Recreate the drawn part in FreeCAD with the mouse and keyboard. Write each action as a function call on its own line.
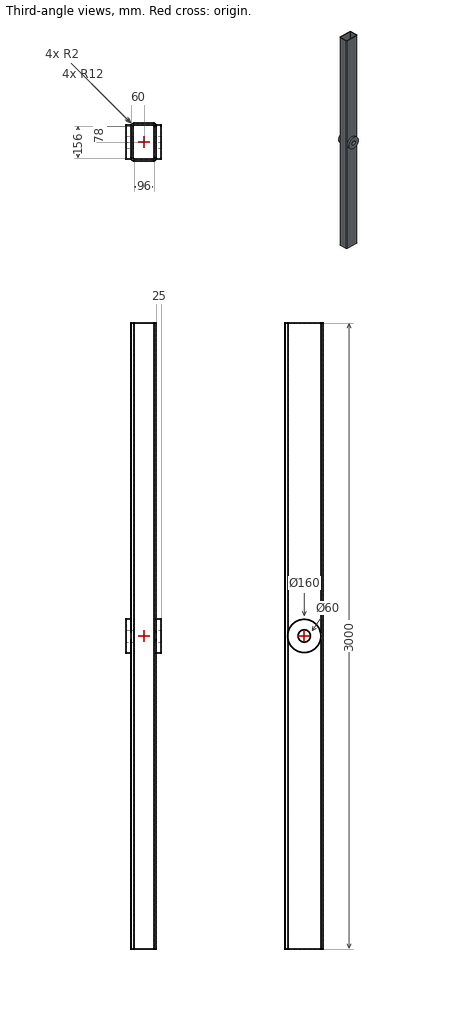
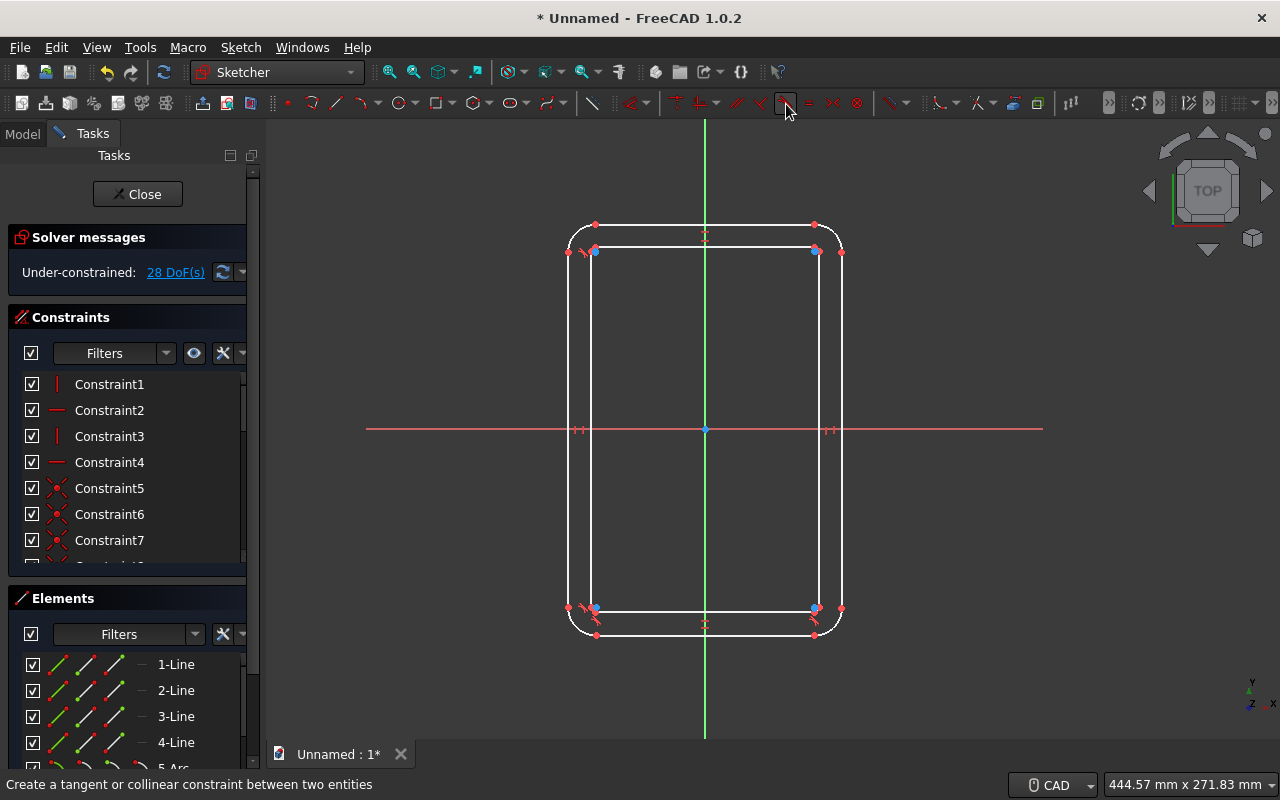
click(842, 502)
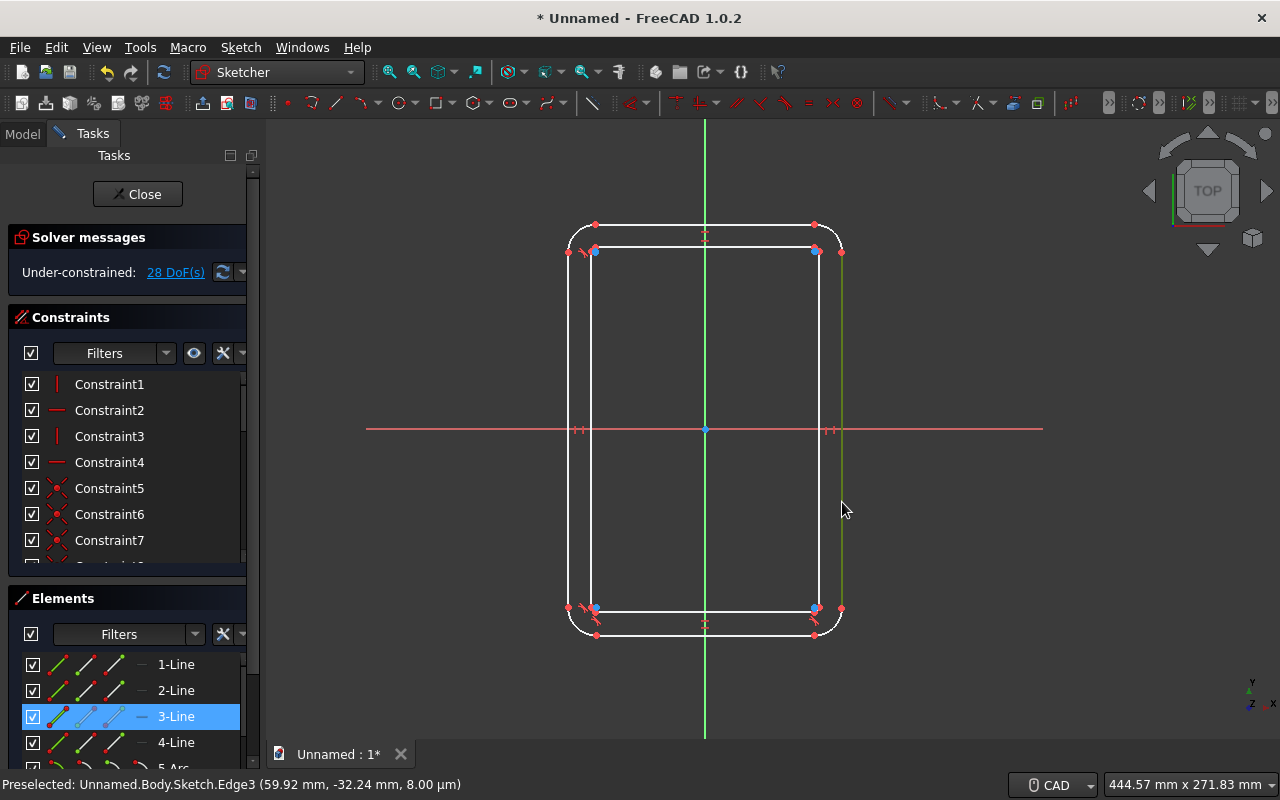
click(827, 633)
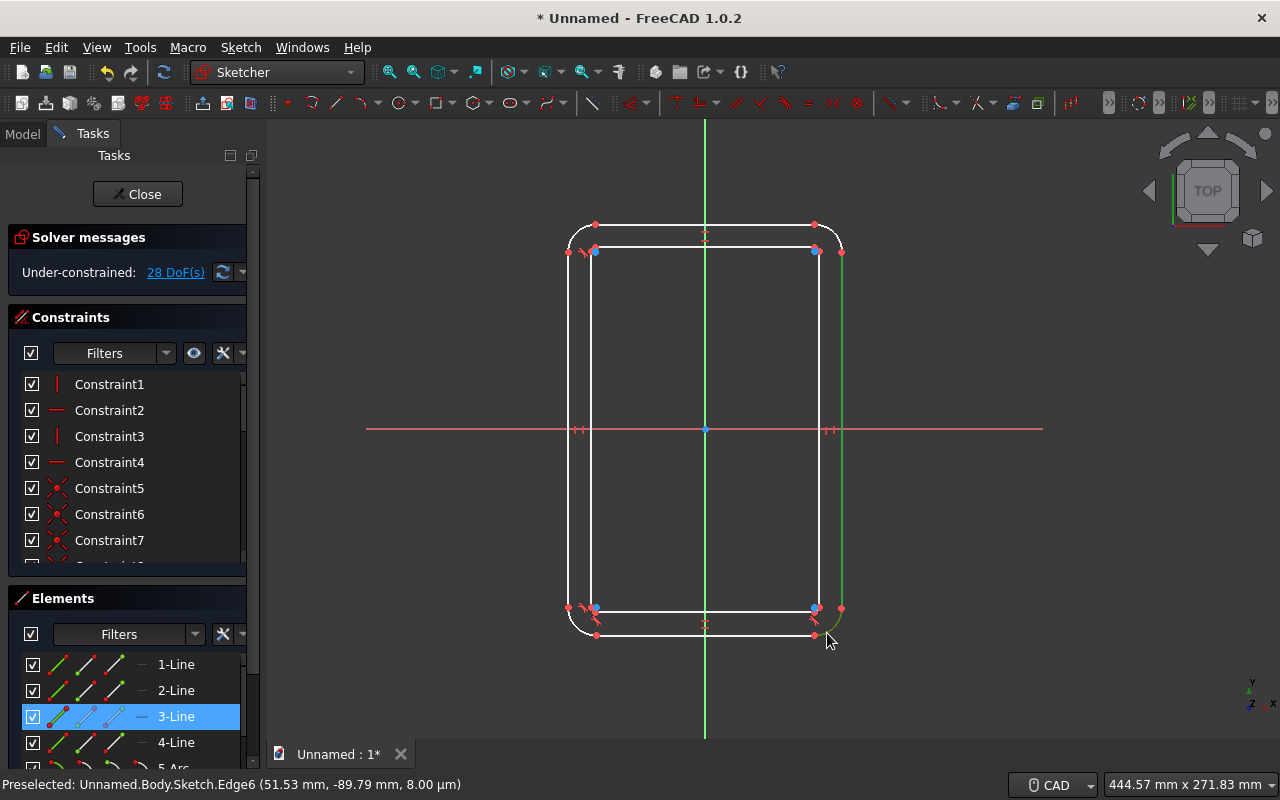
click(786, 104)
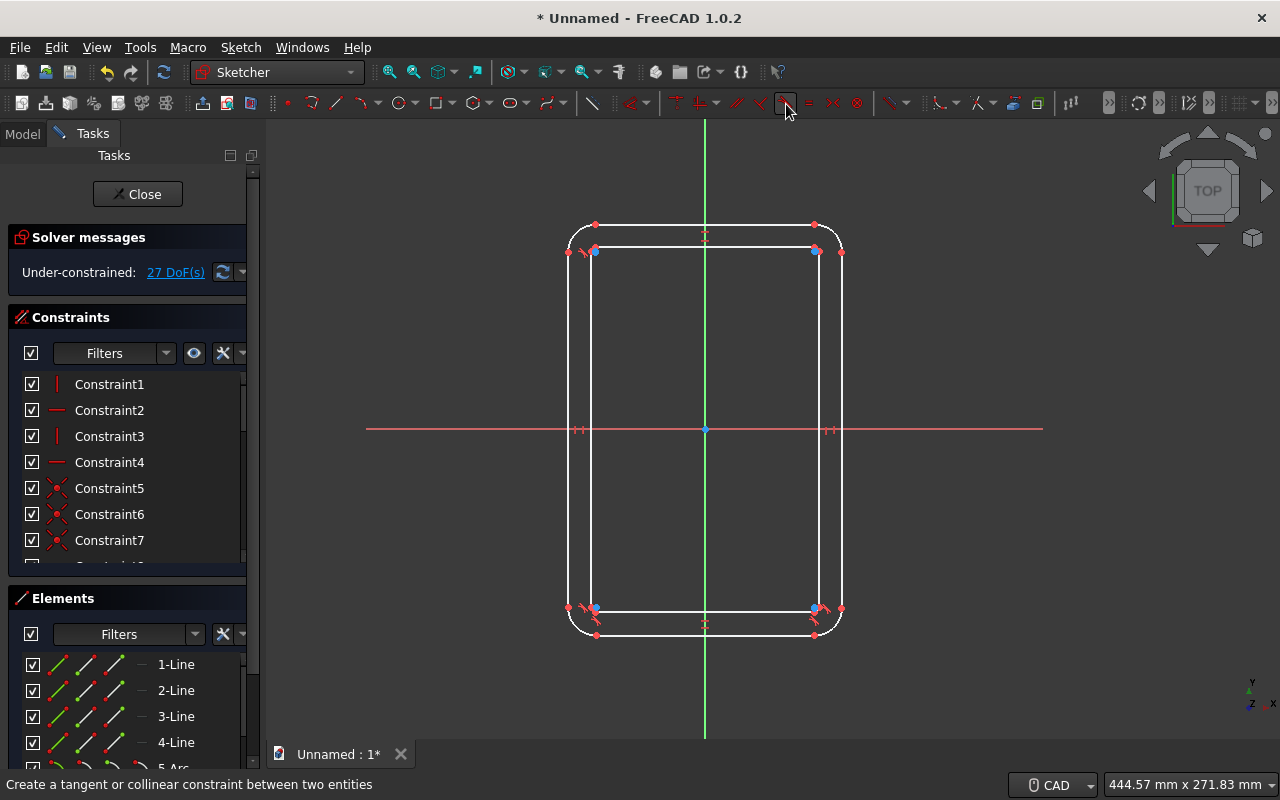
click(842, 501)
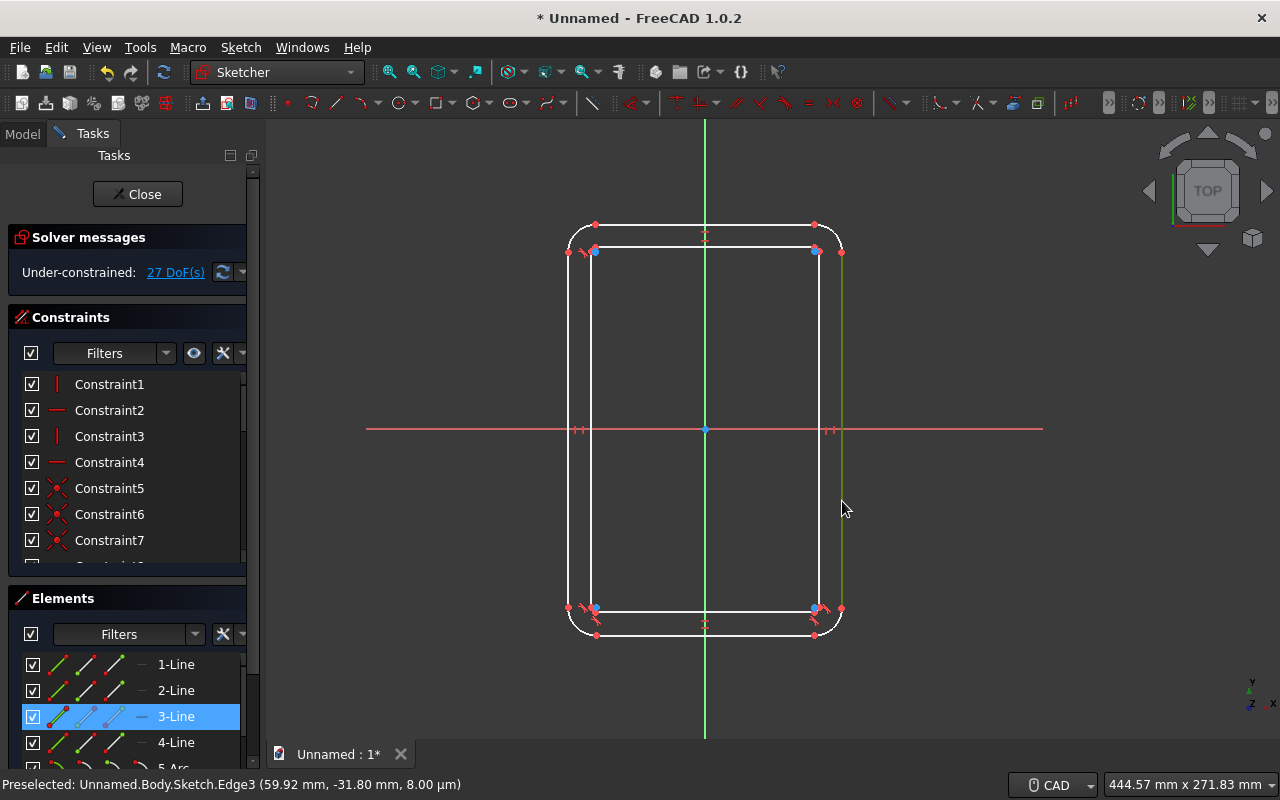
click(839, 240)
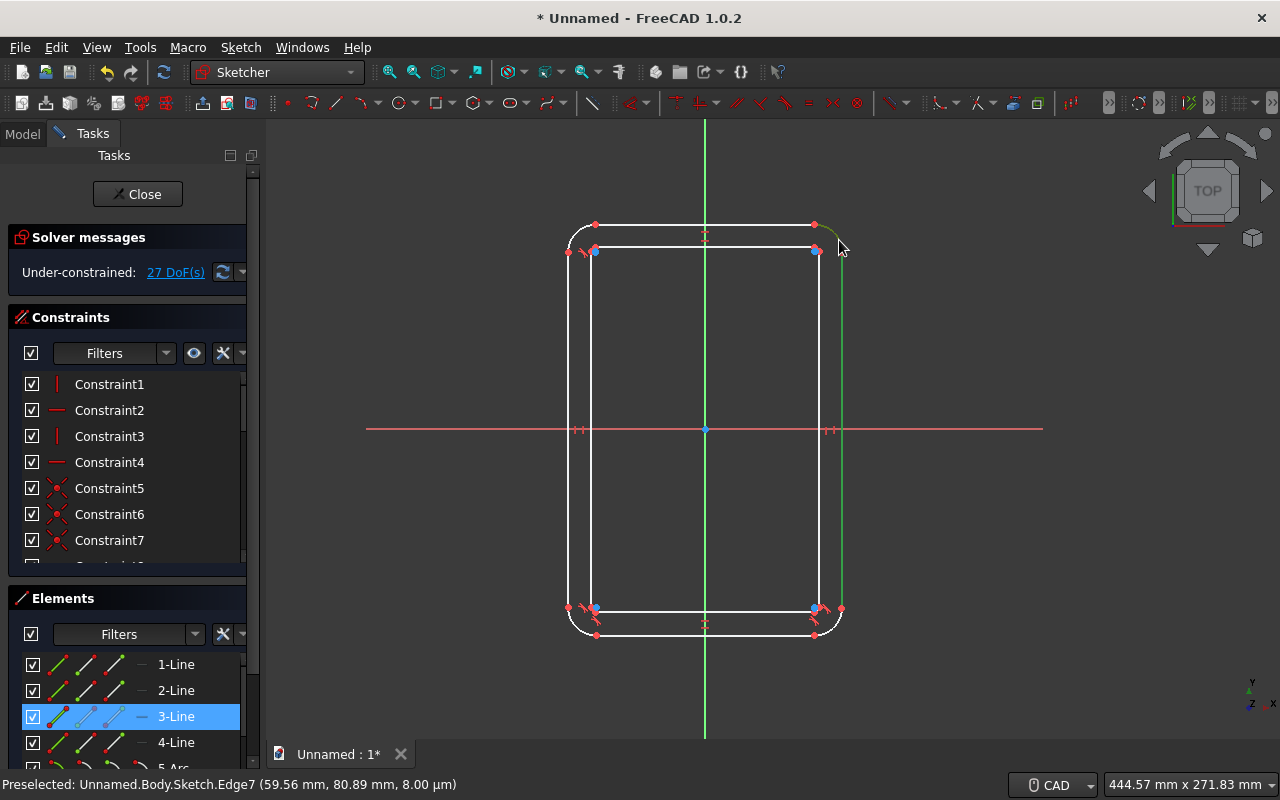
click(786, 104)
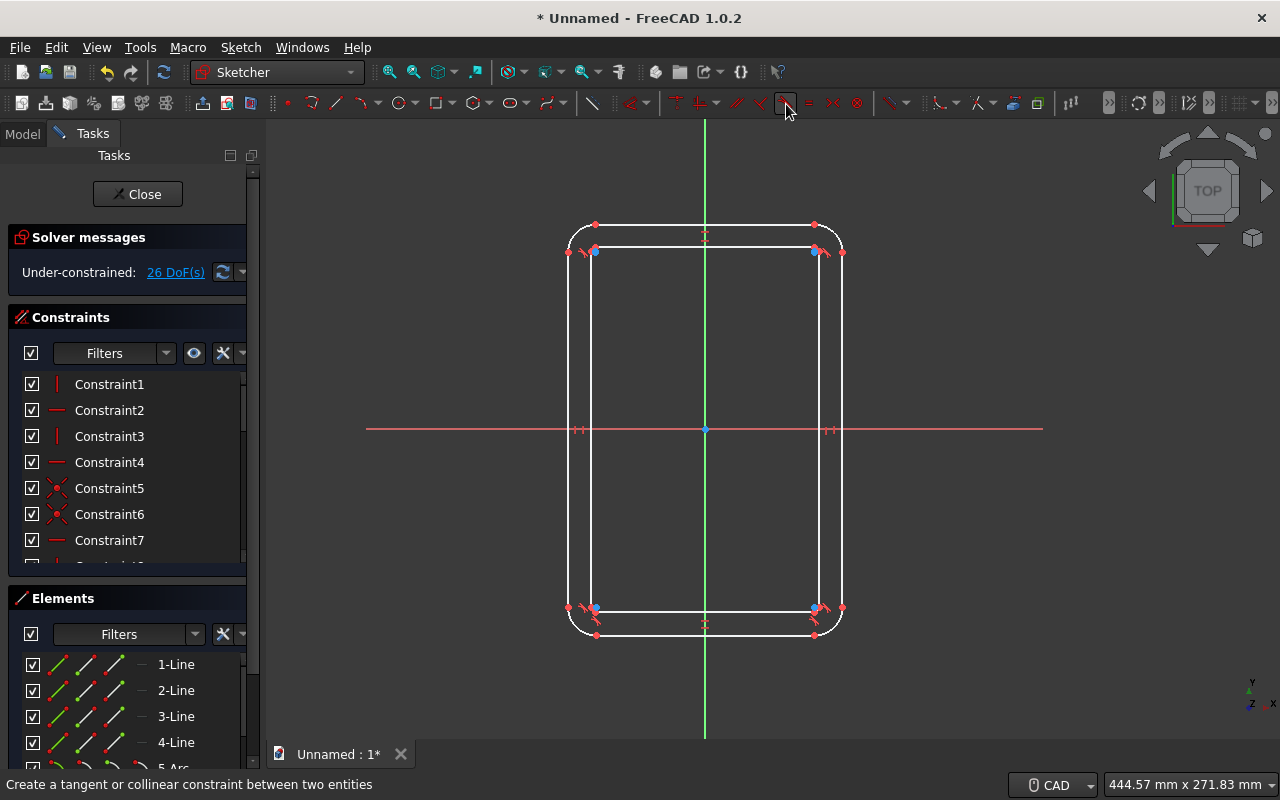
click(749, 225)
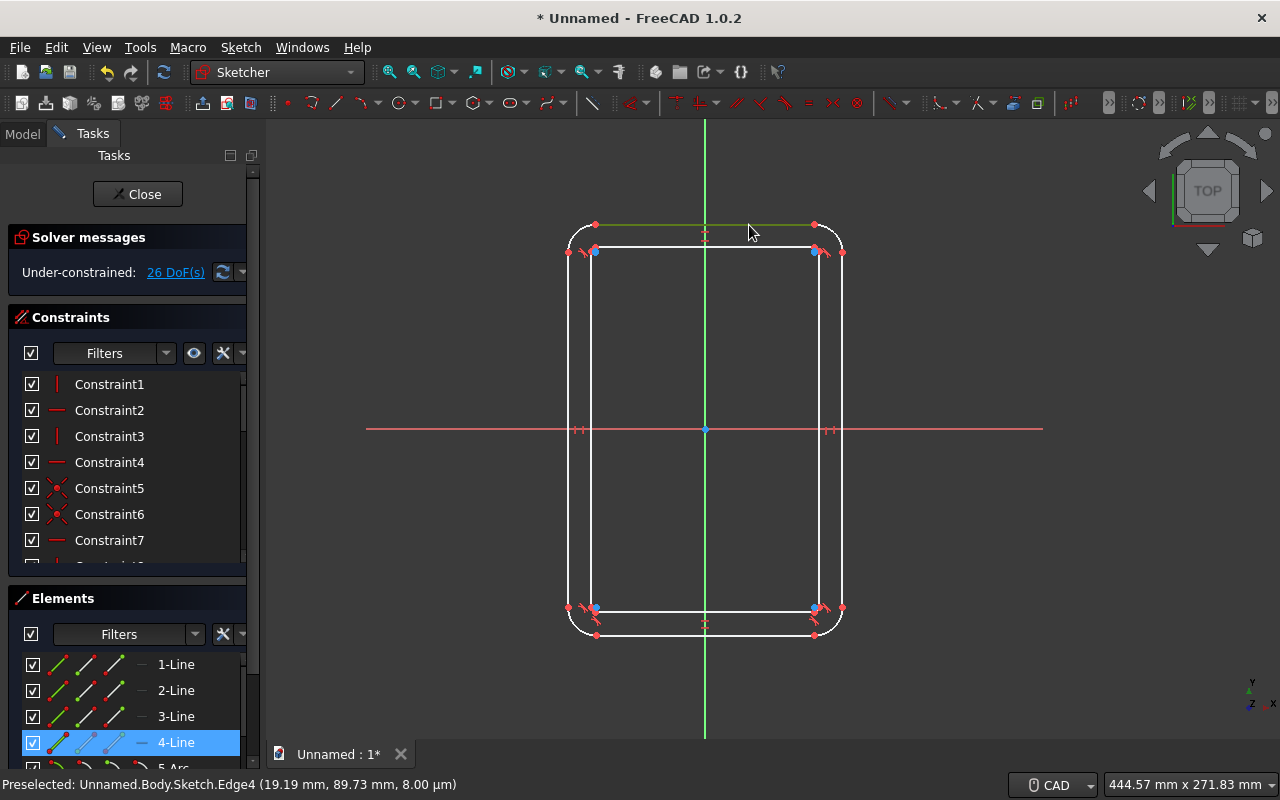
click(839, 240)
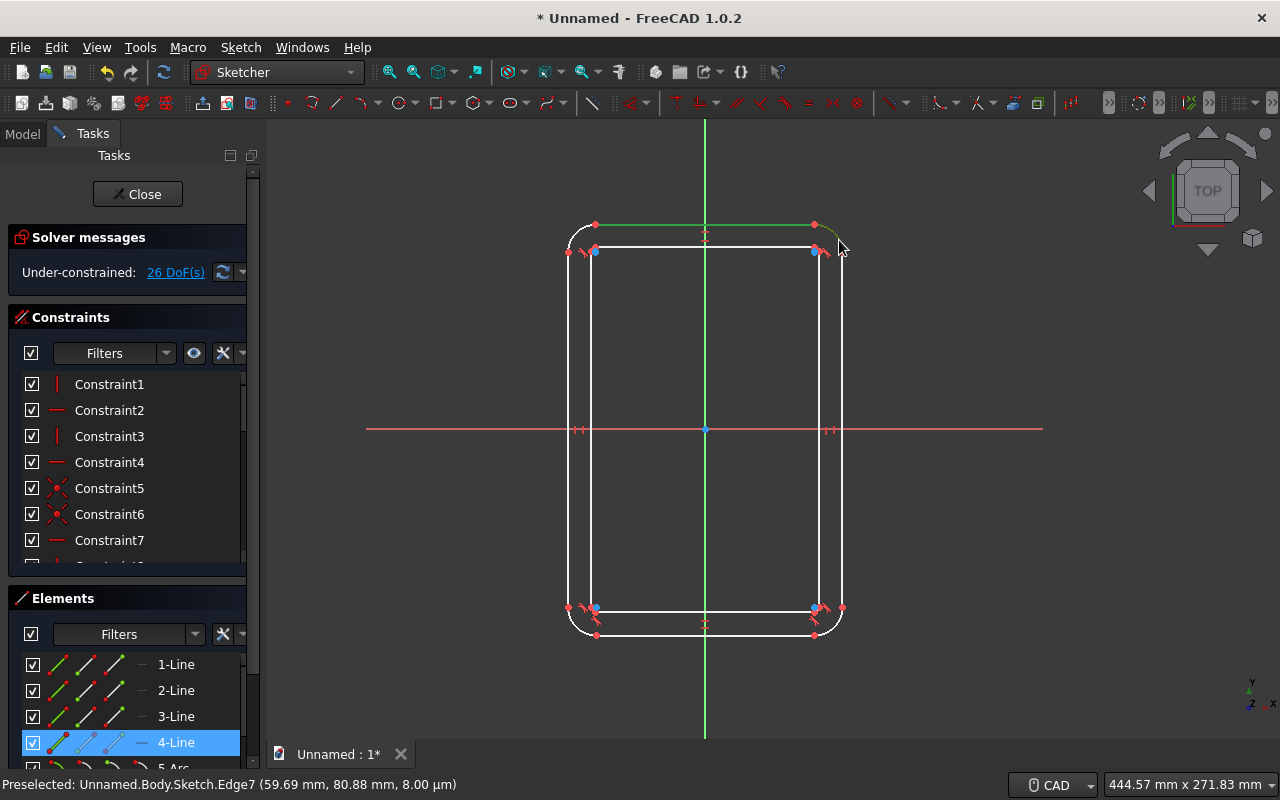
click(786, 104)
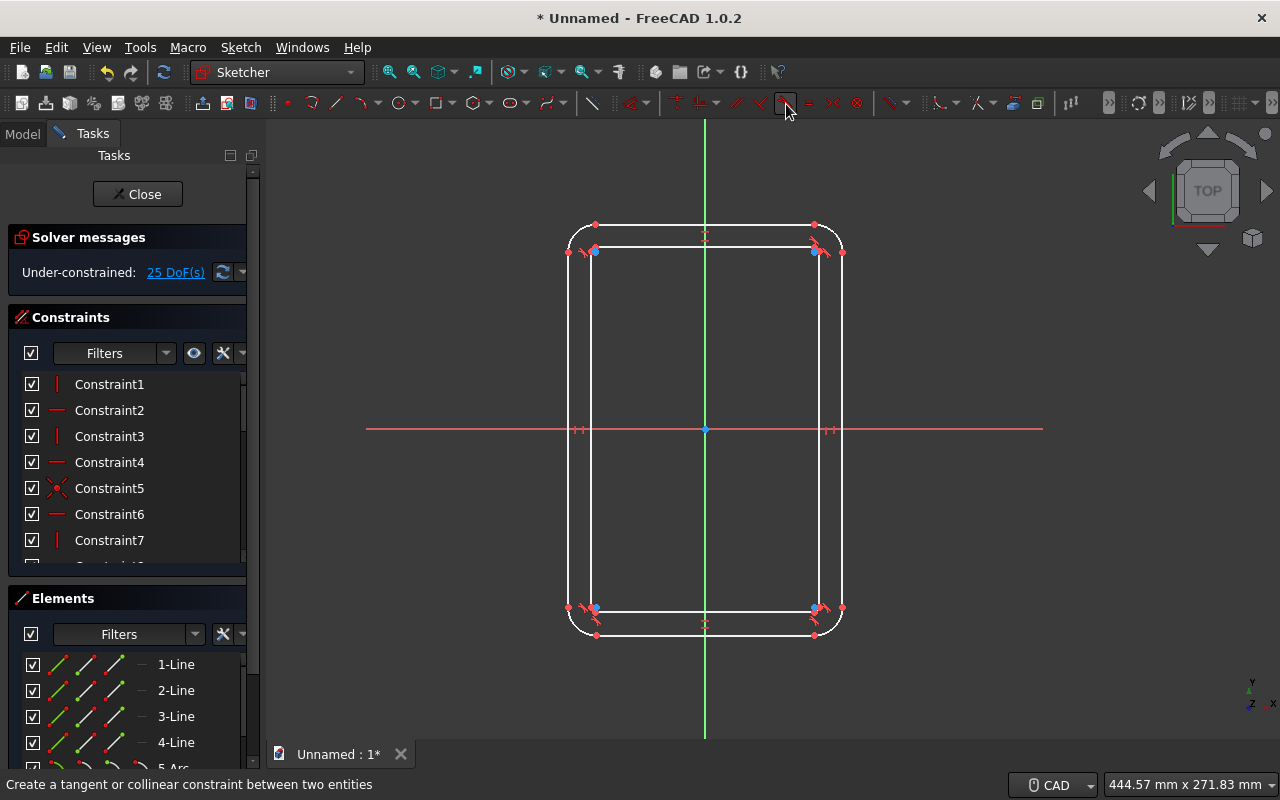
click(749, 225)